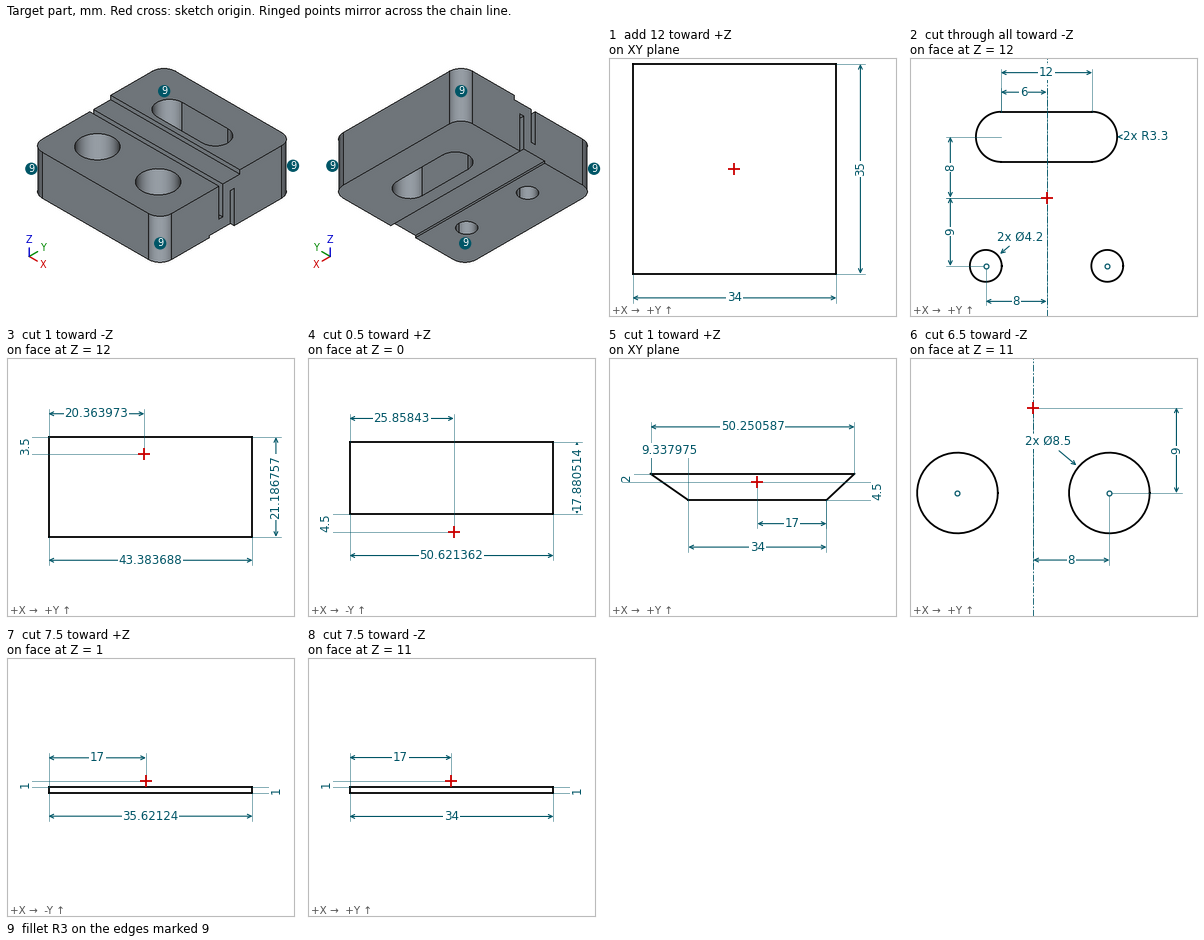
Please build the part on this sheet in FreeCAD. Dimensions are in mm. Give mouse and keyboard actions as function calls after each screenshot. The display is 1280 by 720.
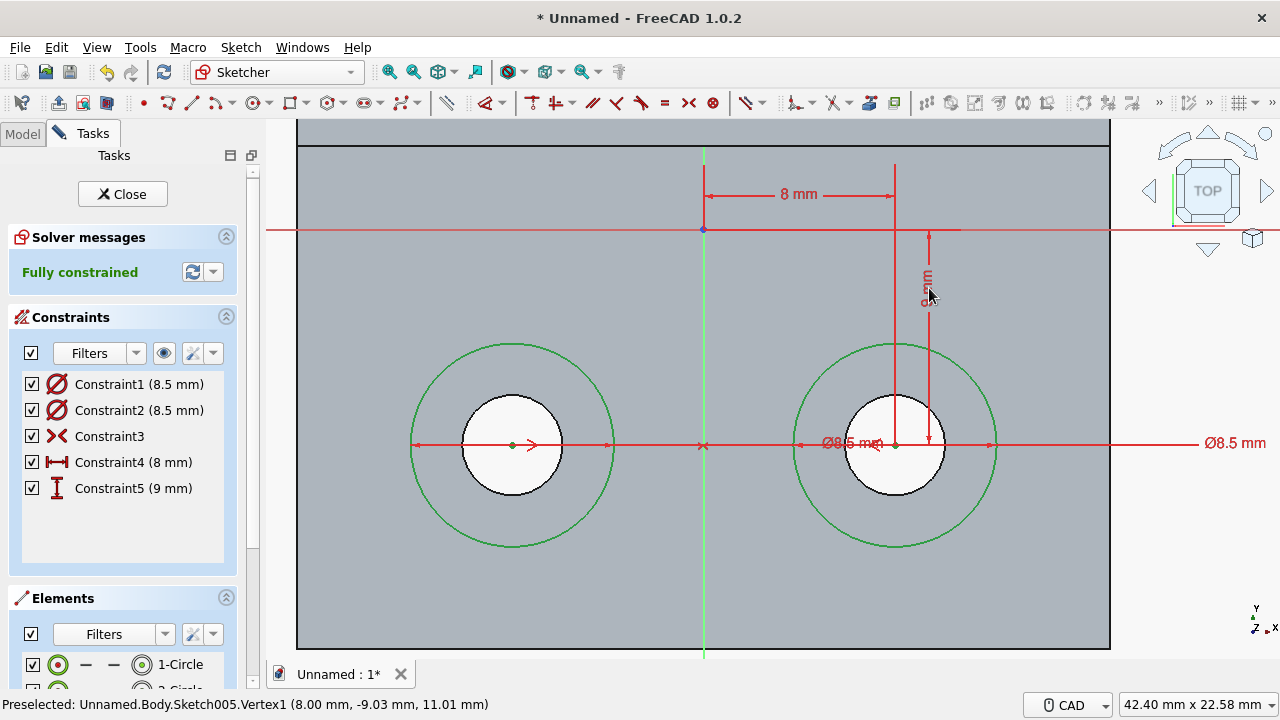
click(123, 194)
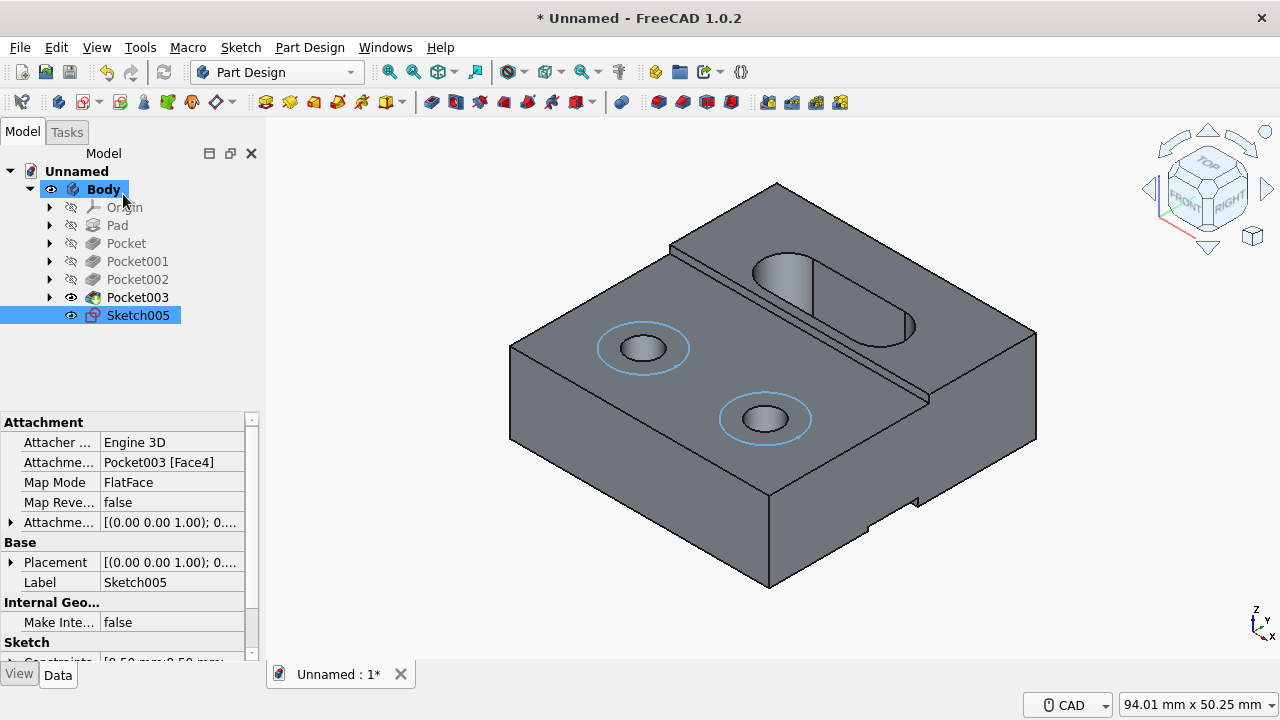
click(432, 102)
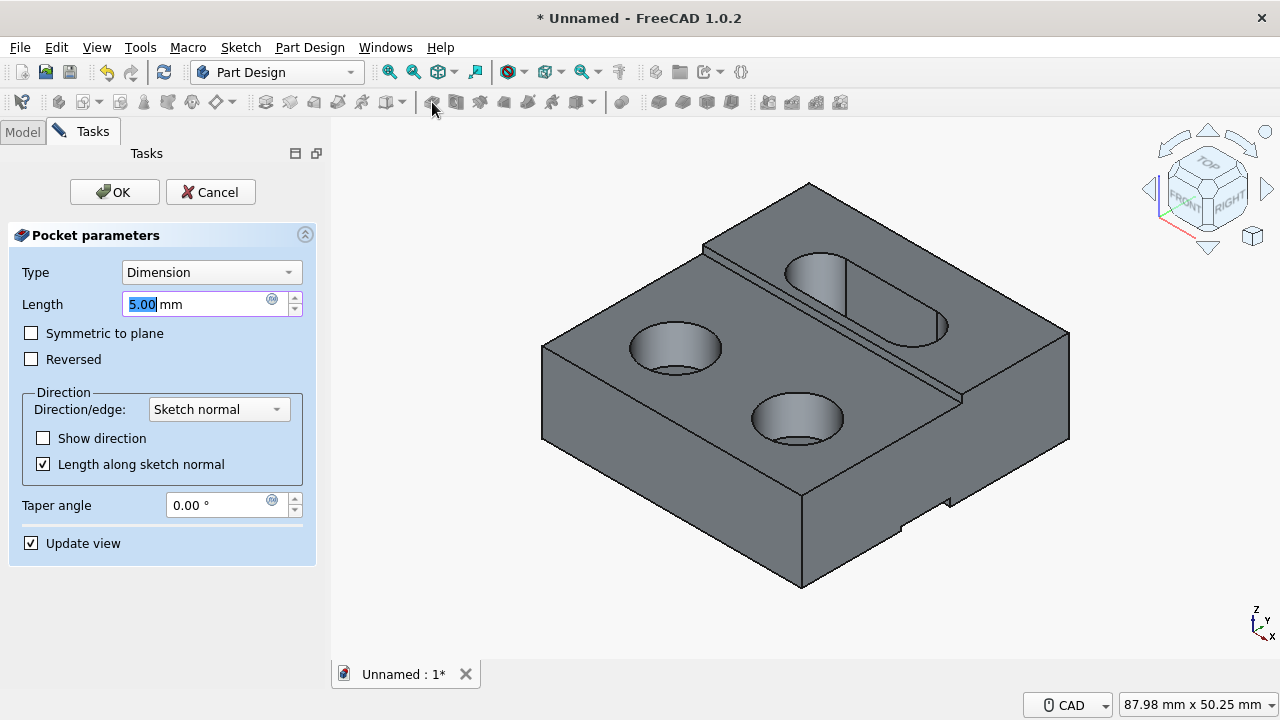
text(6.5)
key(Tab)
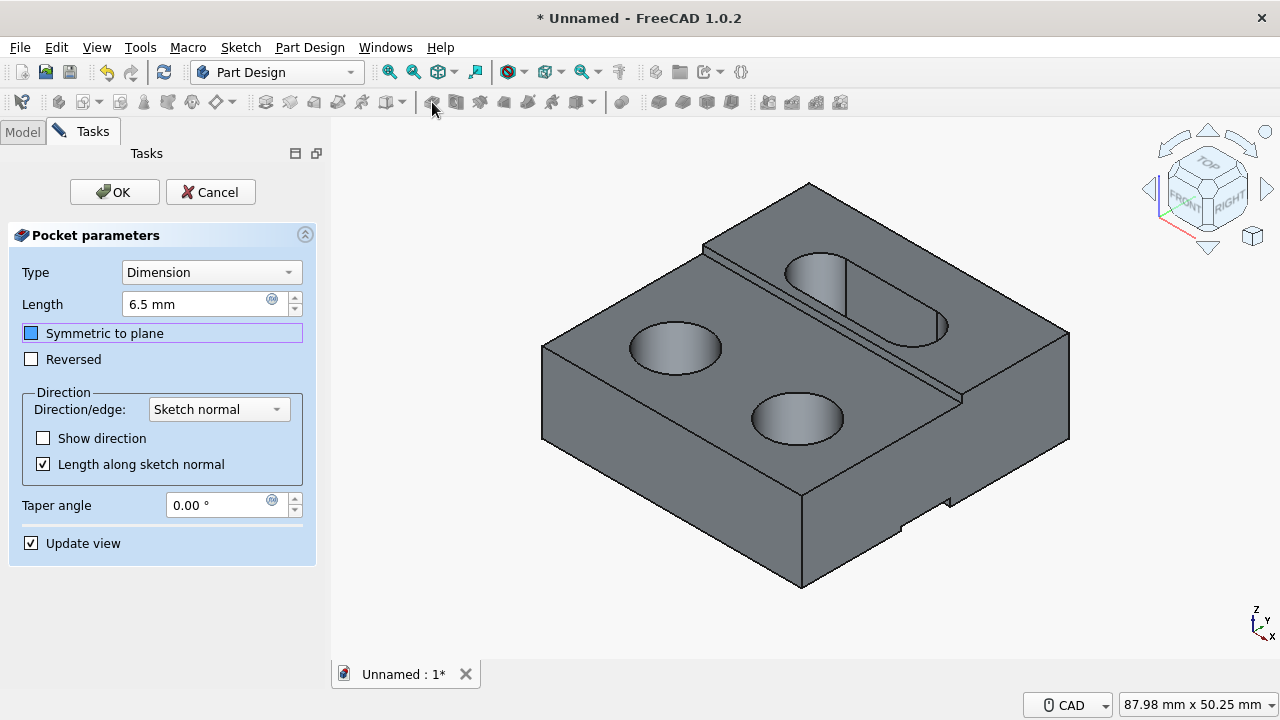
click(115, 192)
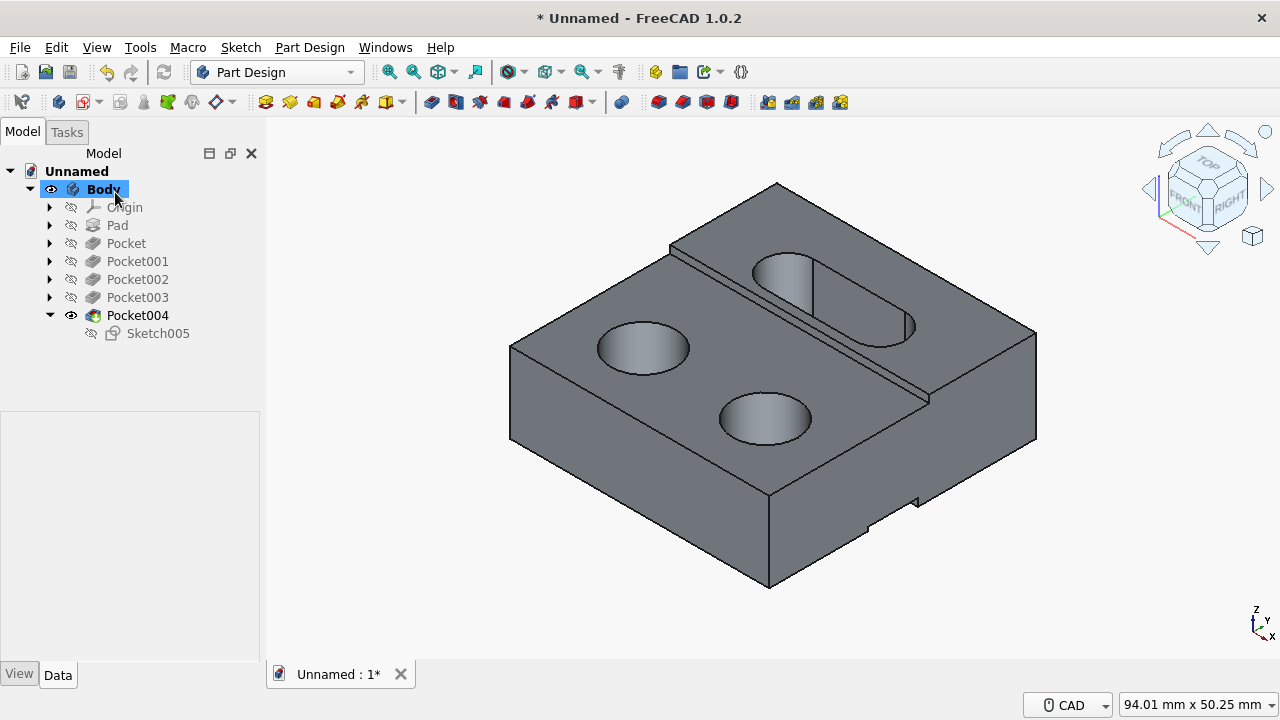
key(5)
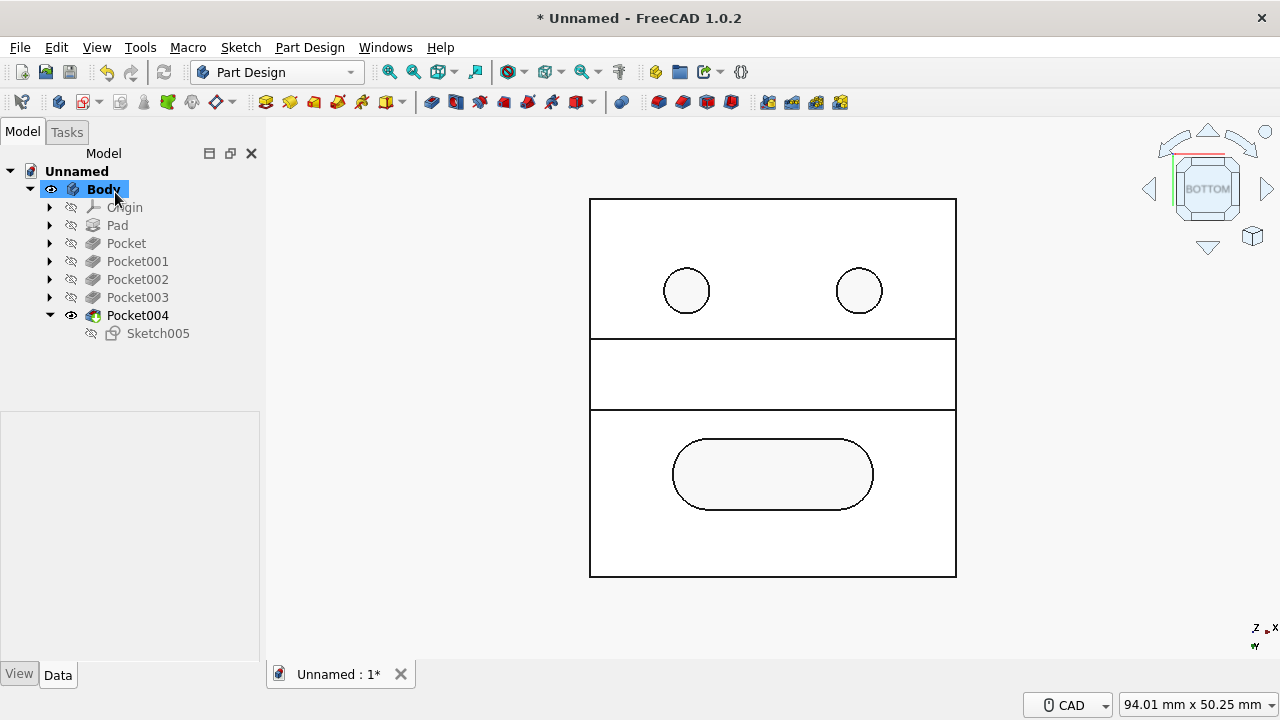
click(878, 374)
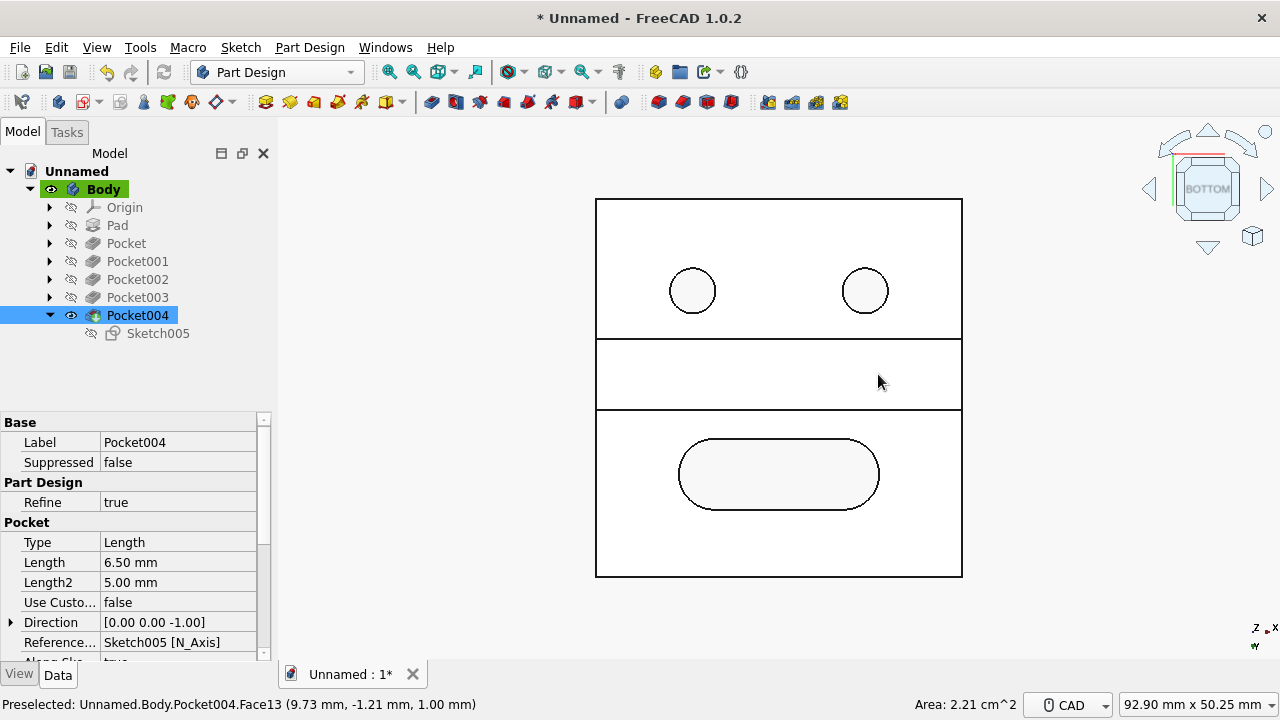
click(84, 102)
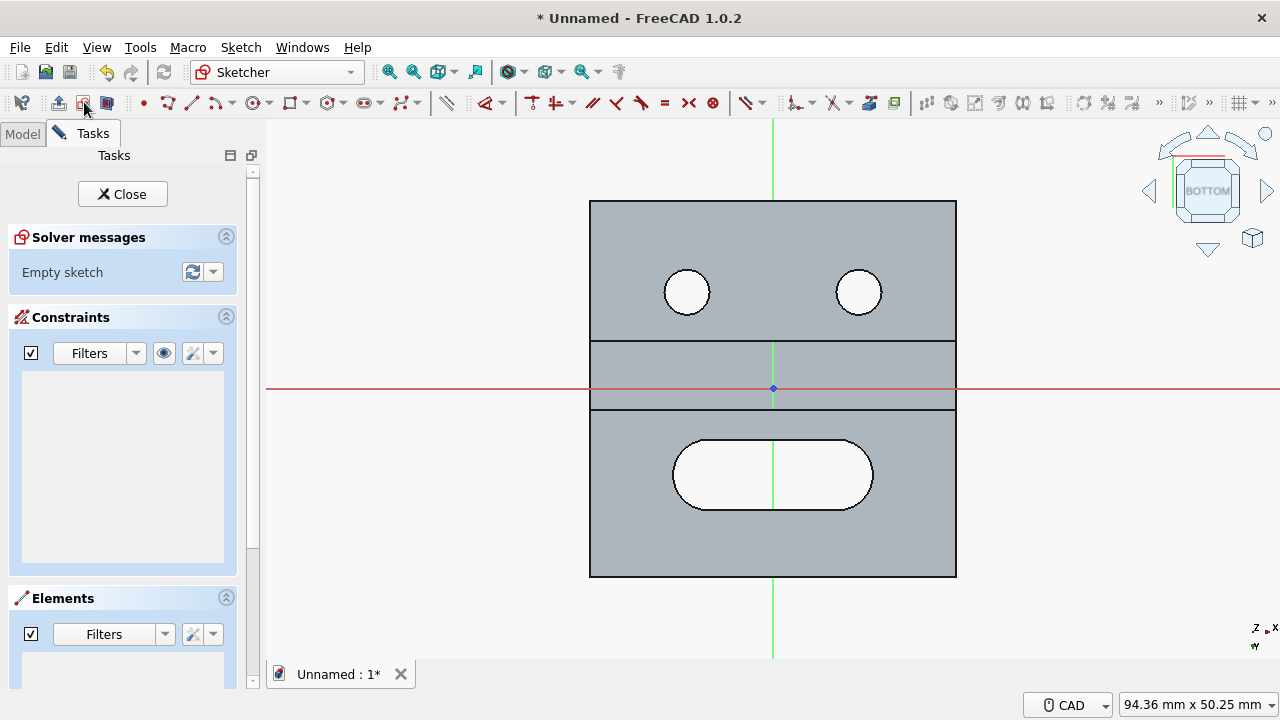
scroll(939, 422, up, 2)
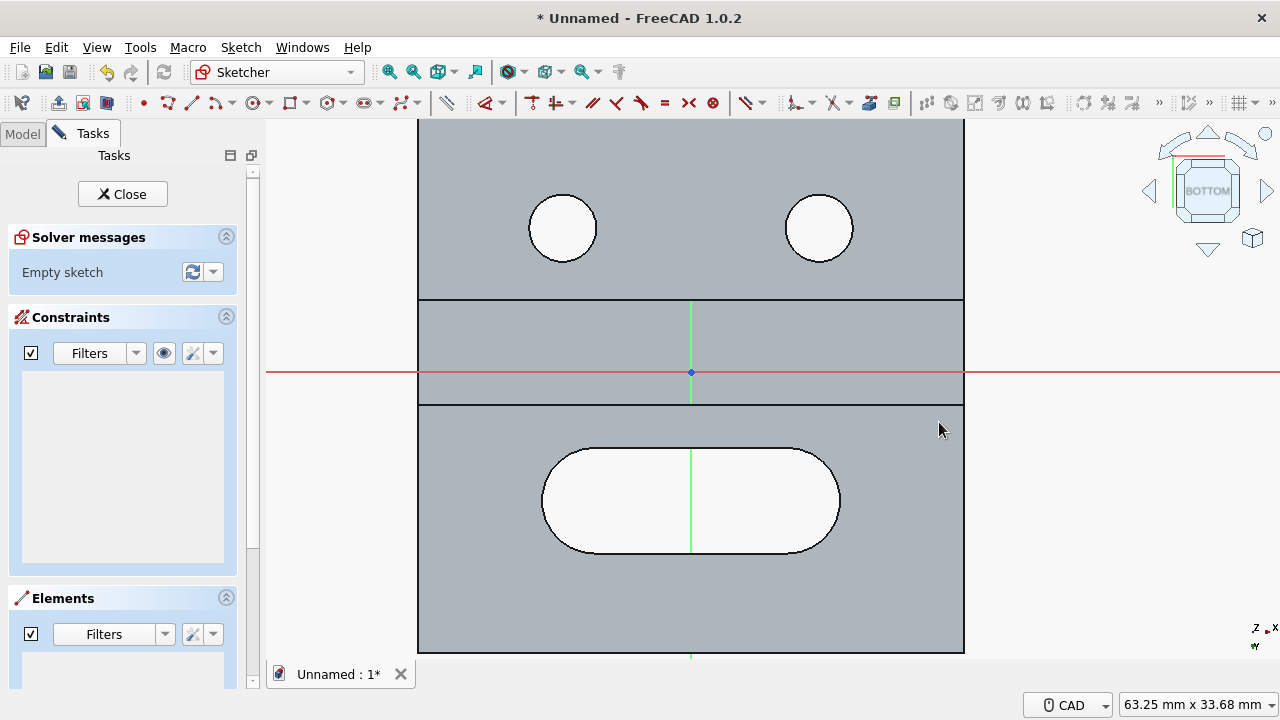
key(g)
key(r)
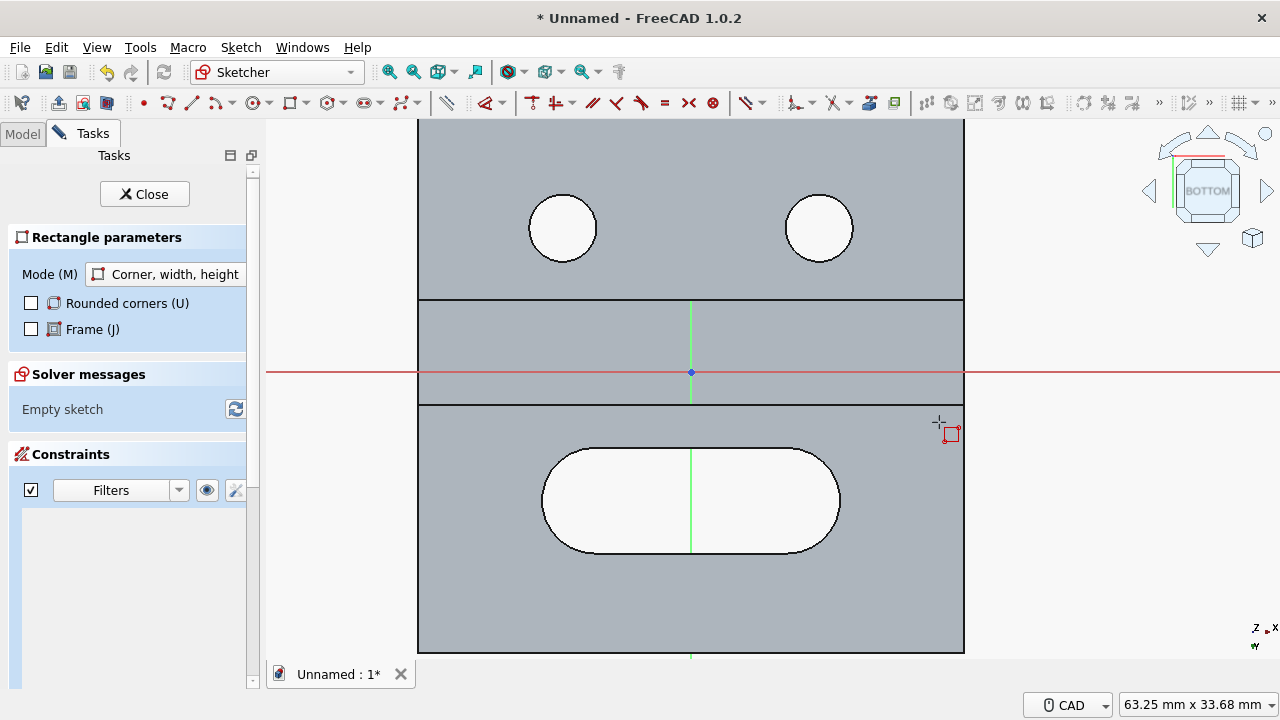
click(418, 389)
move(990, 405)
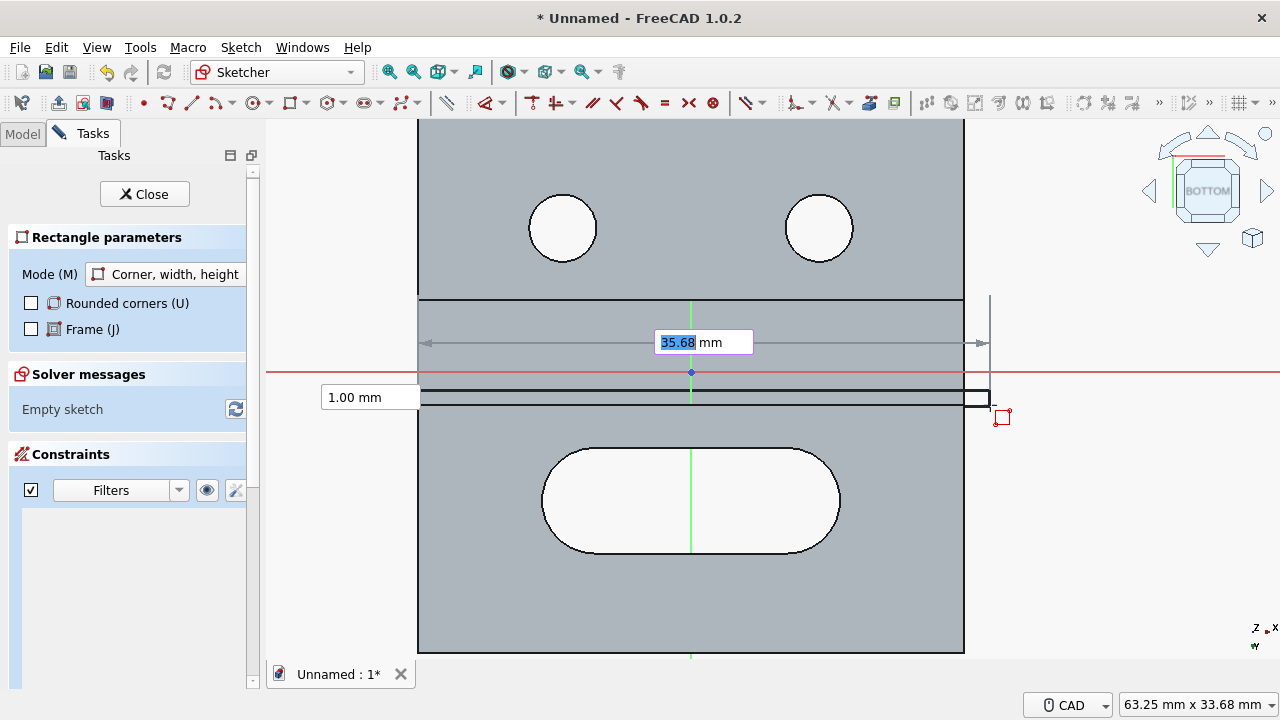
text(35.62124)
key(Tab)
text(1)
key(Return)
key(Escape)